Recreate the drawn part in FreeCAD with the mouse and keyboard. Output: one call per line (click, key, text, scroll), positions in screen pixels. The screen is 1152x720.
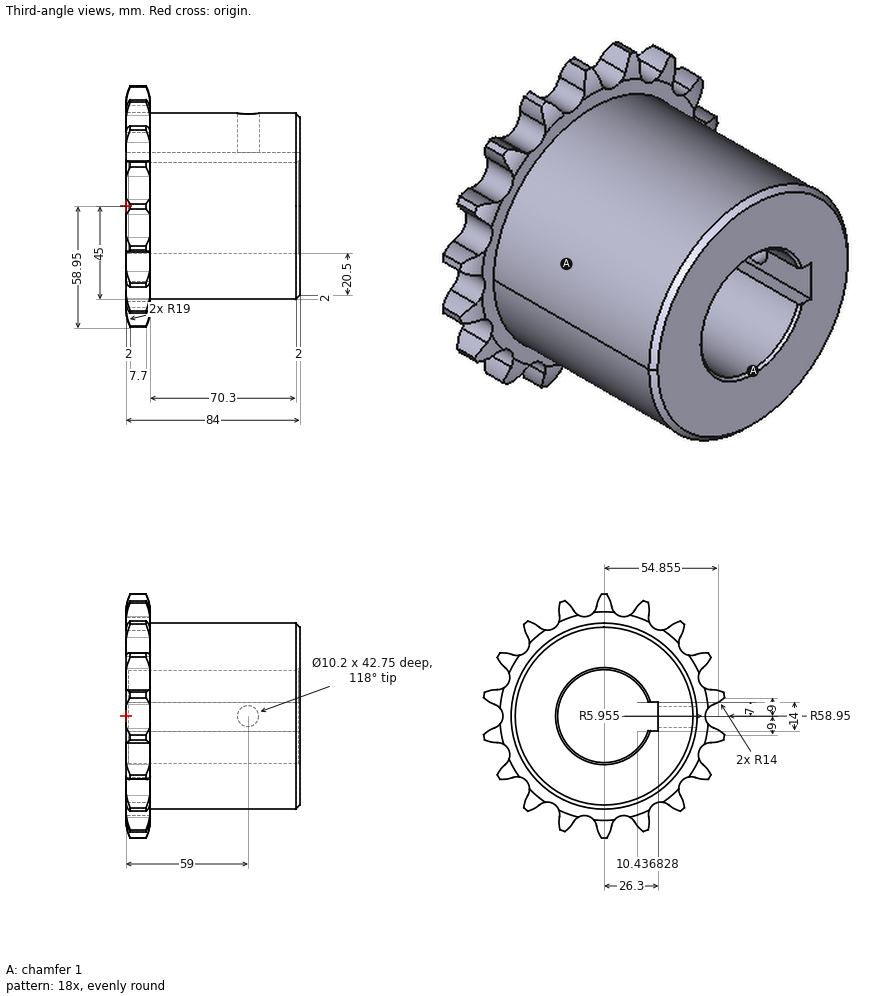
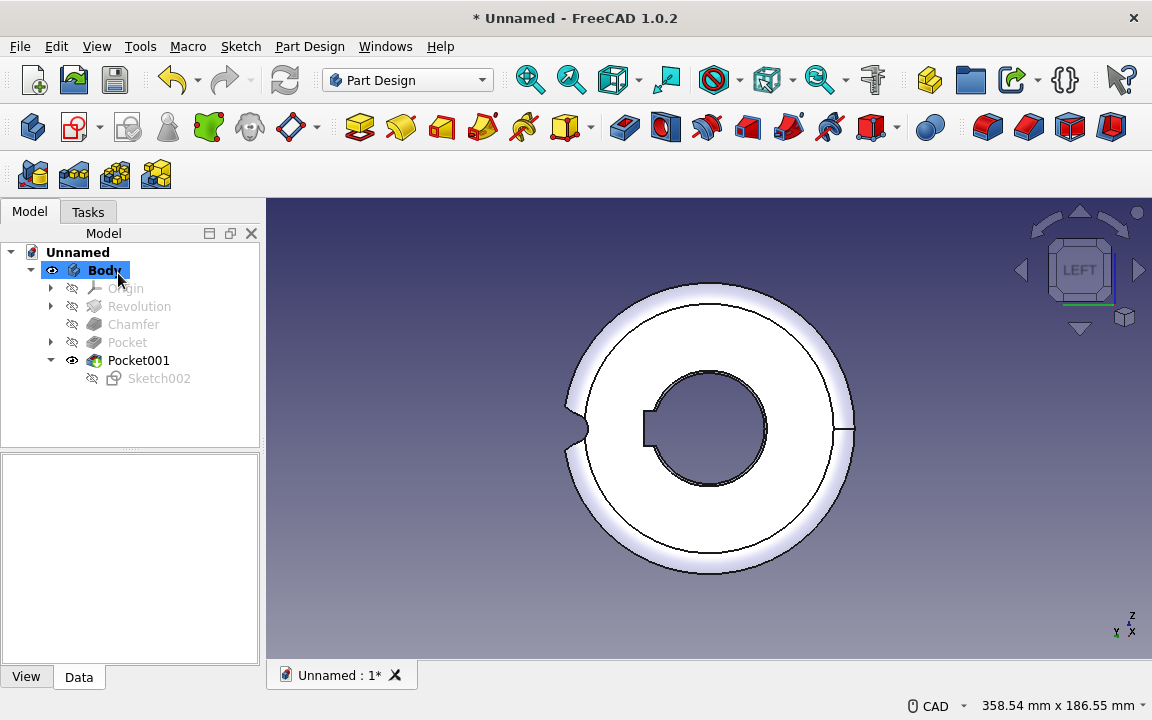
click(117, 360)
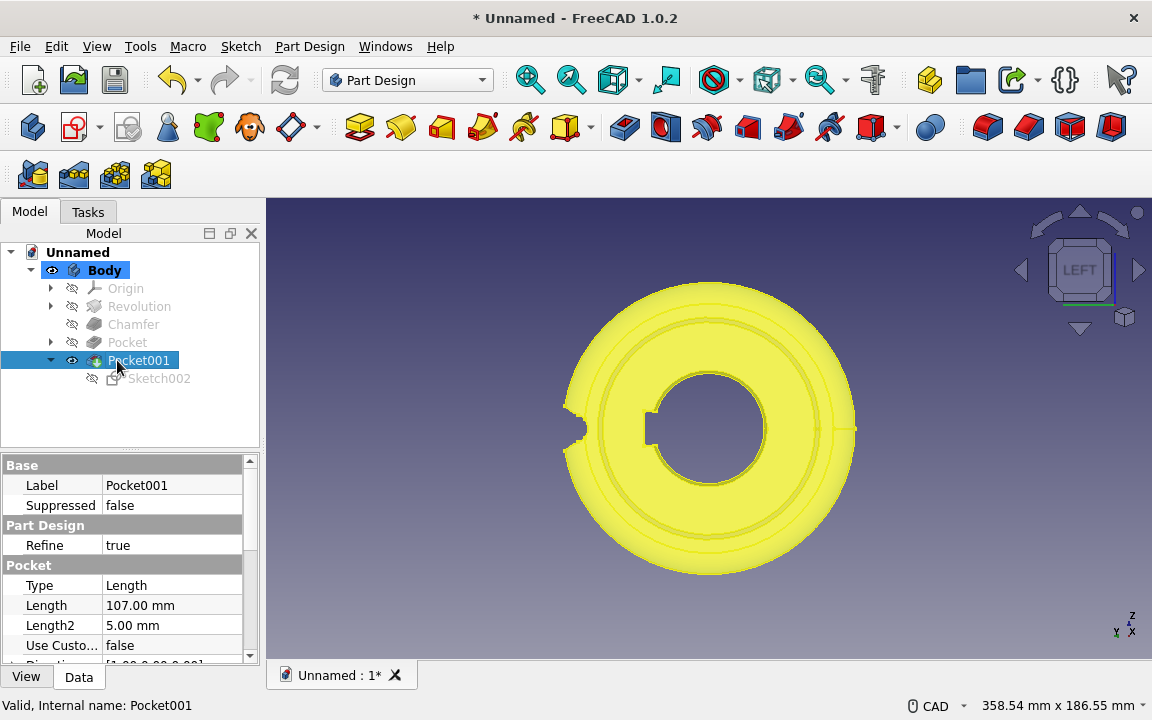
click(115, 174)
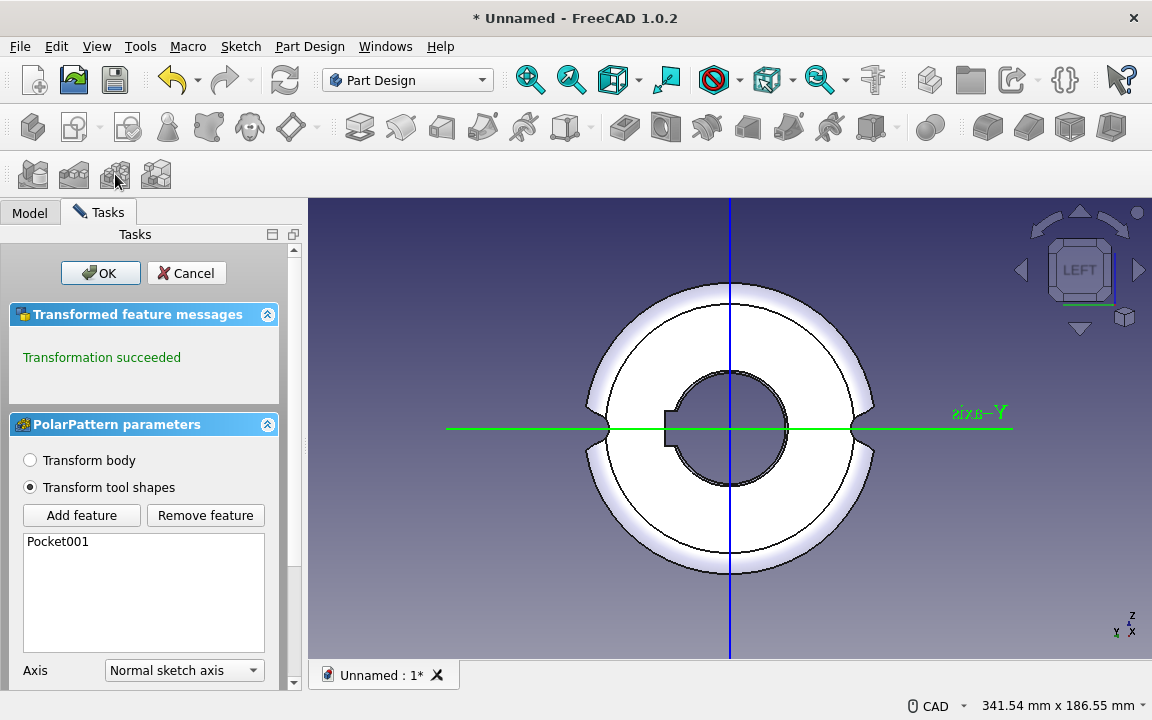
click(185, 670)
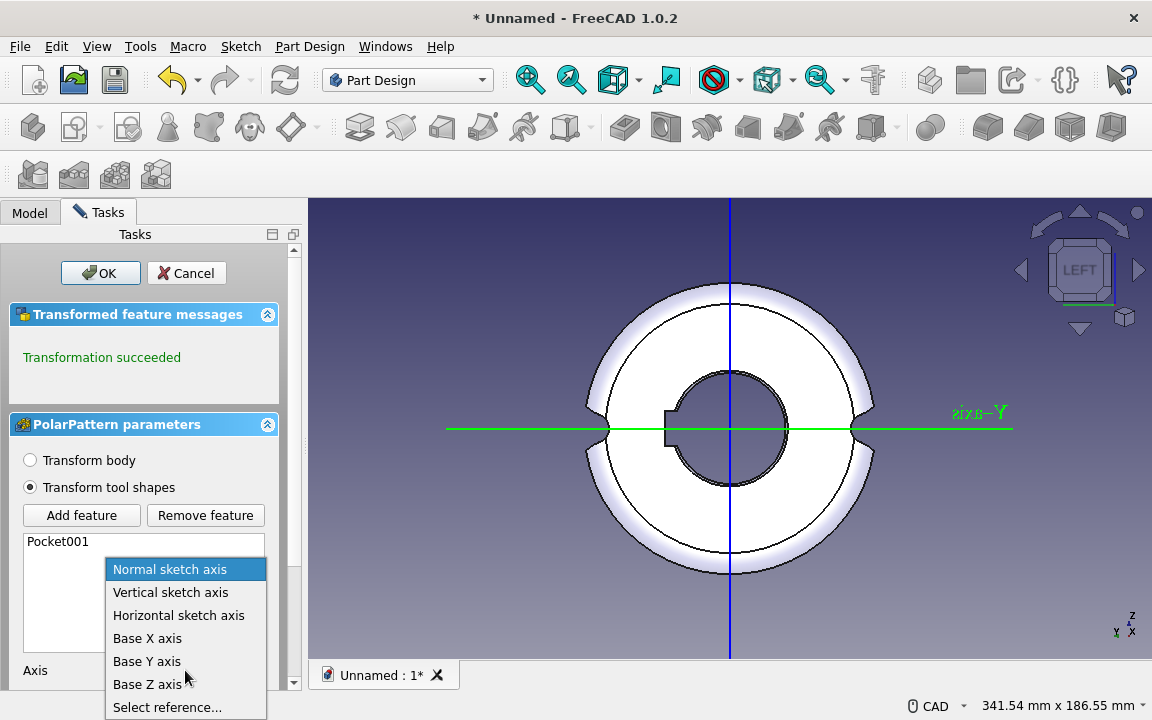
click(184, 638)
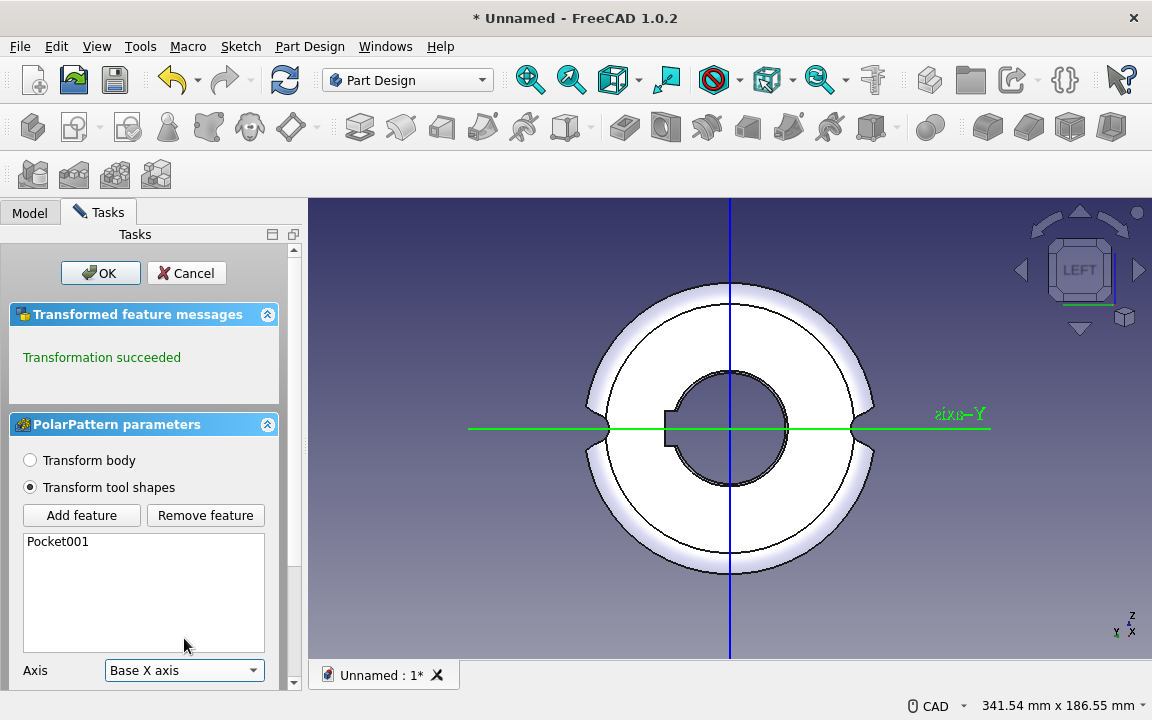
scroll(294, 467, down, 3)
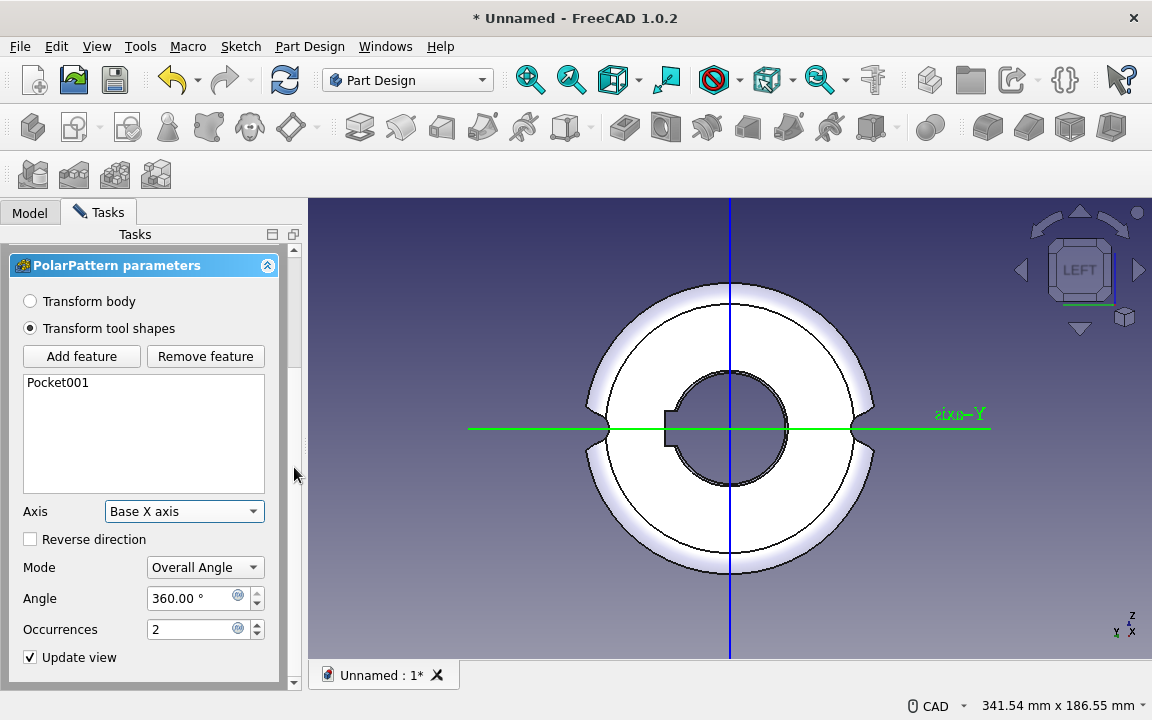
triple_click(199, 630)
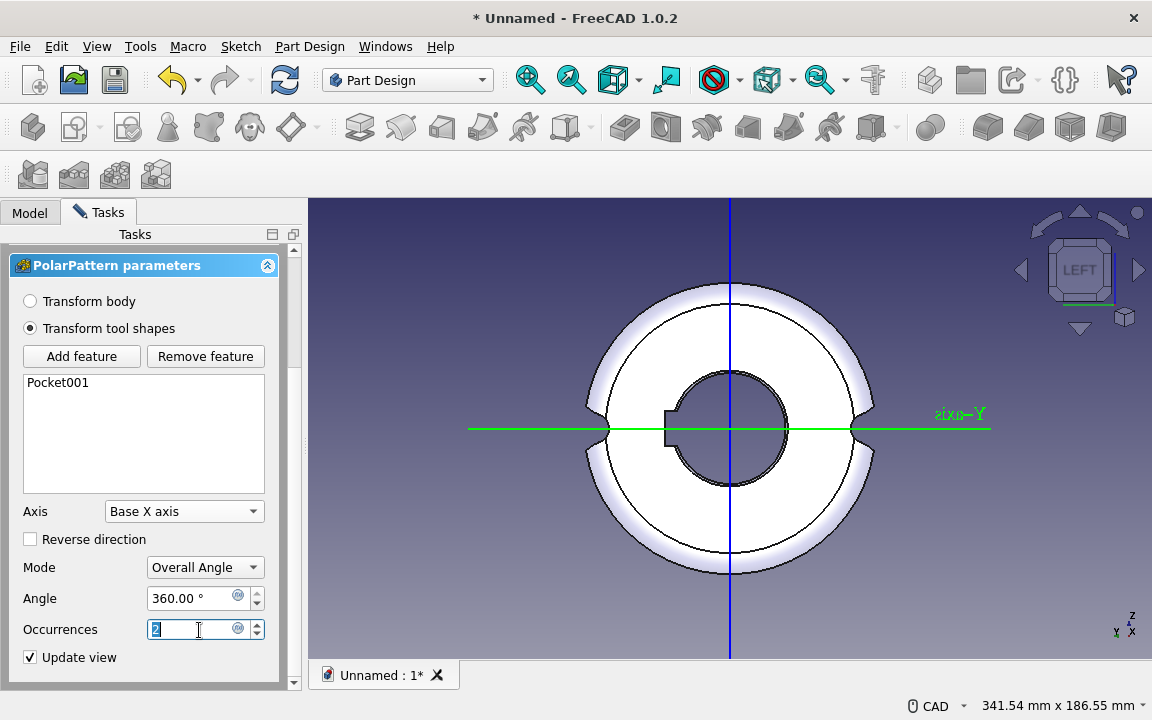
text(18)
key(Tab)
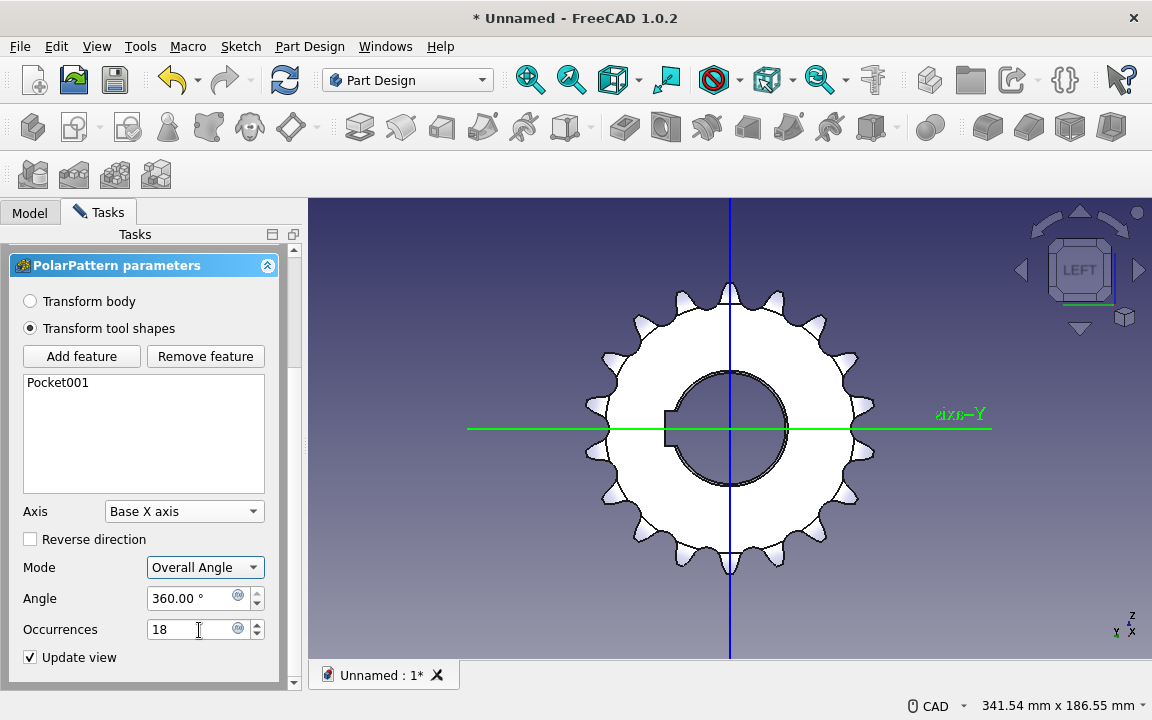
scroll(294, 467, up, 4)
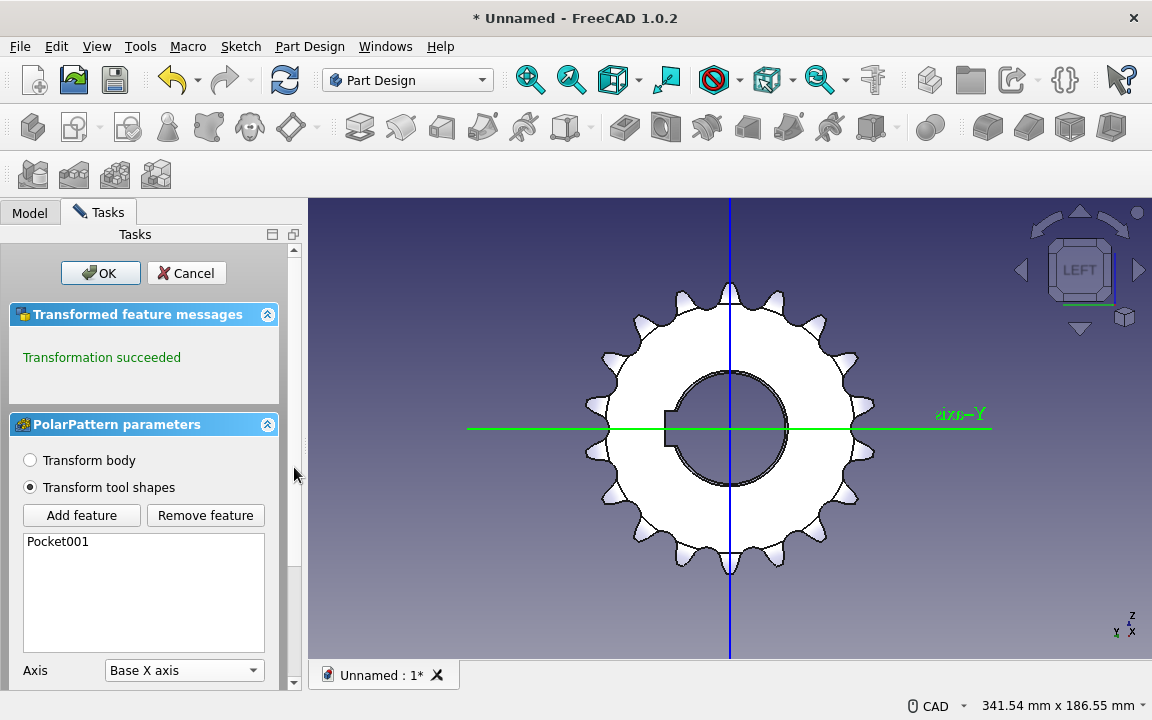
click(101, 273)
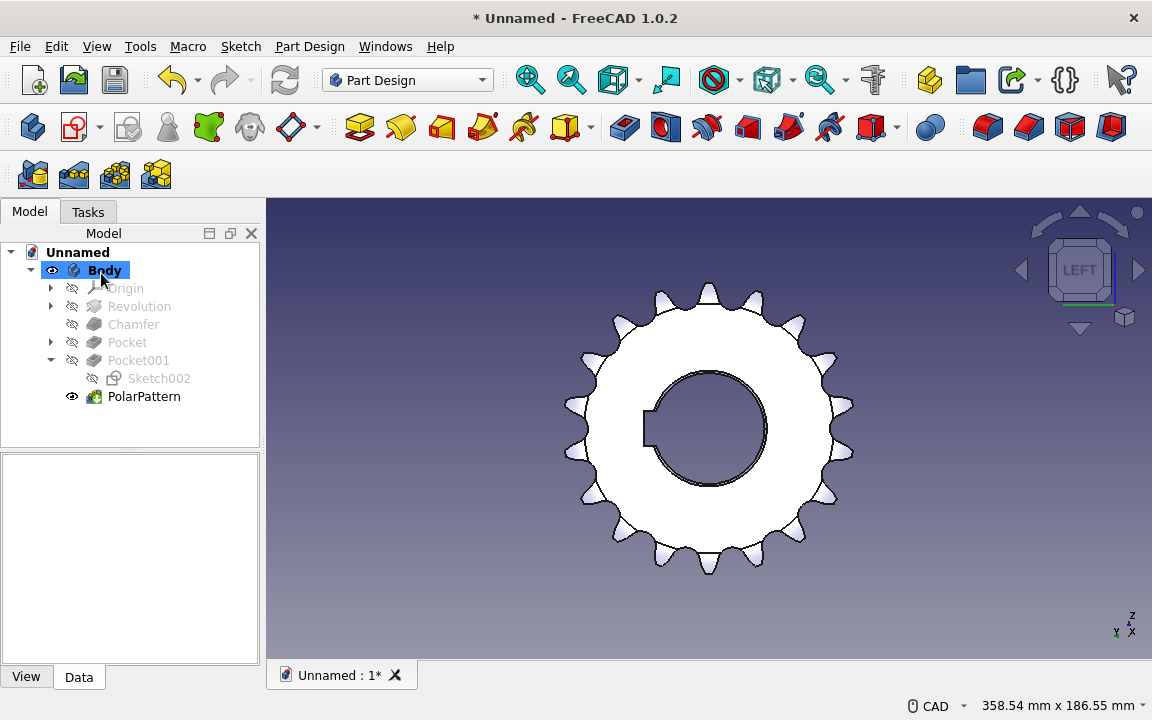
click(51, 288)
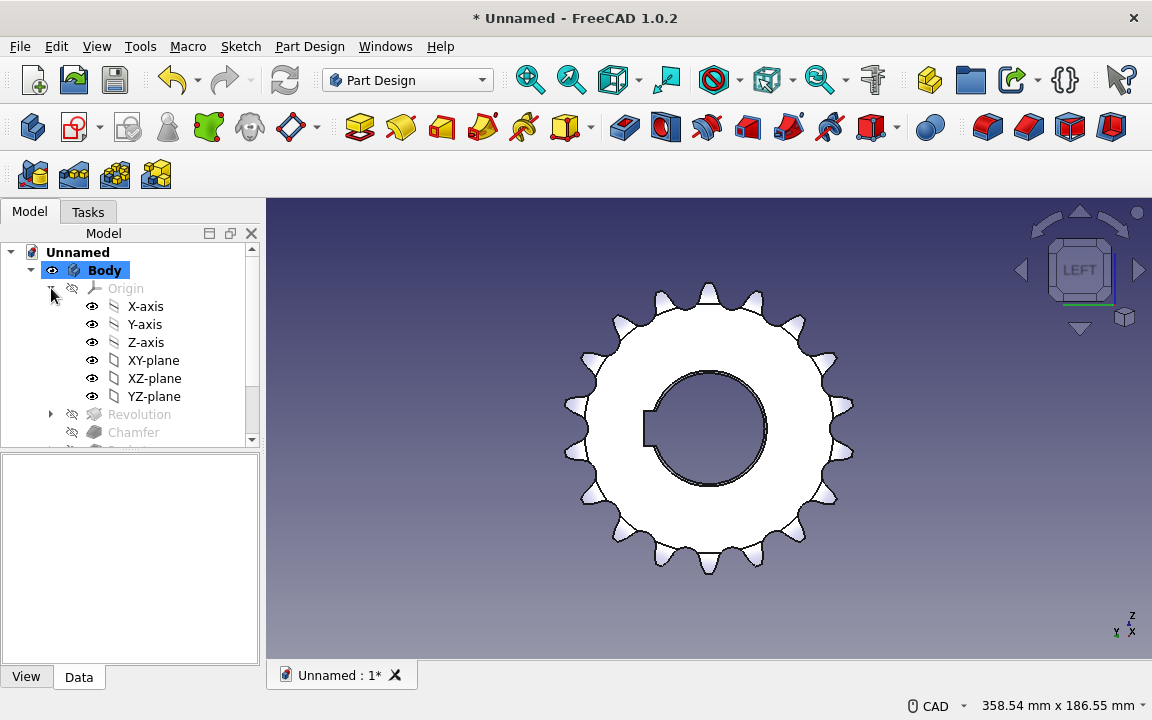
click(137, 378)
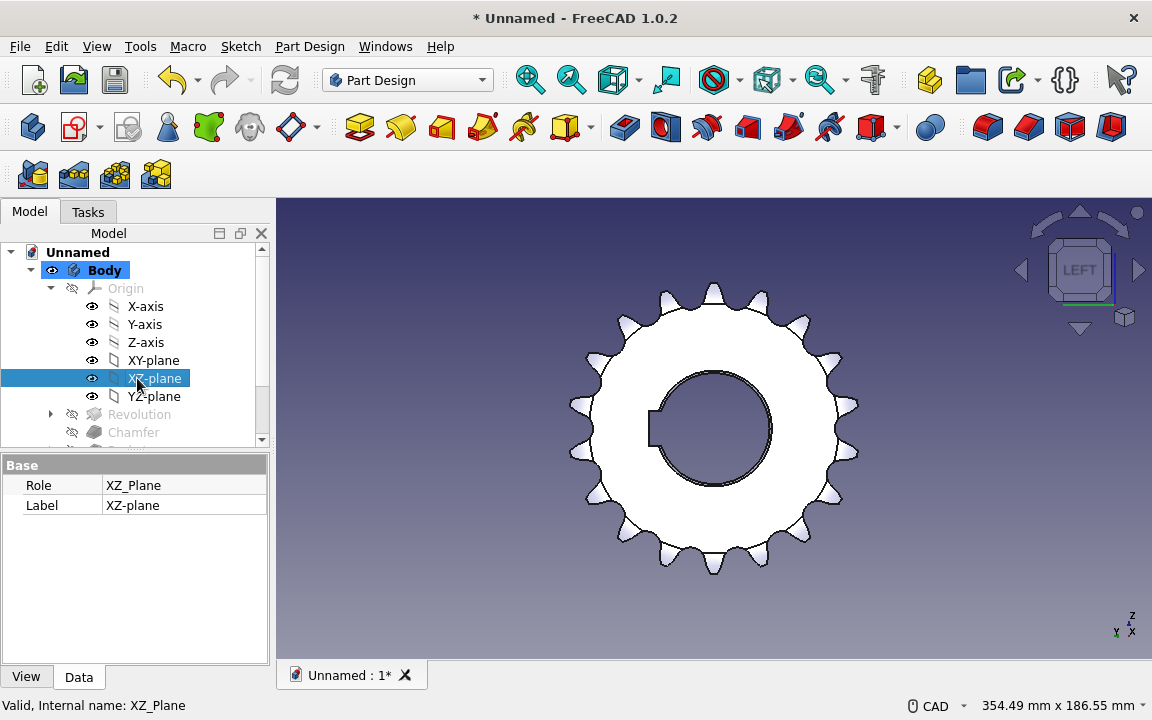
click(290, 128)